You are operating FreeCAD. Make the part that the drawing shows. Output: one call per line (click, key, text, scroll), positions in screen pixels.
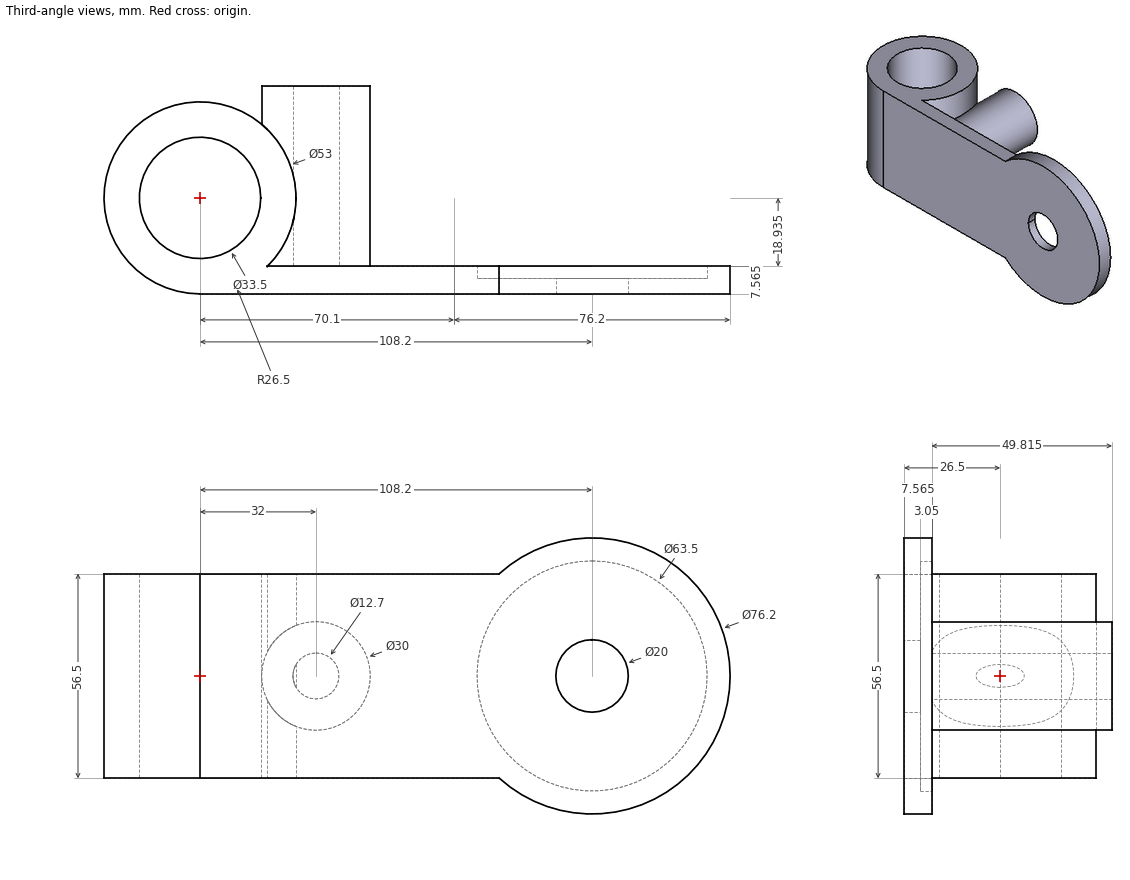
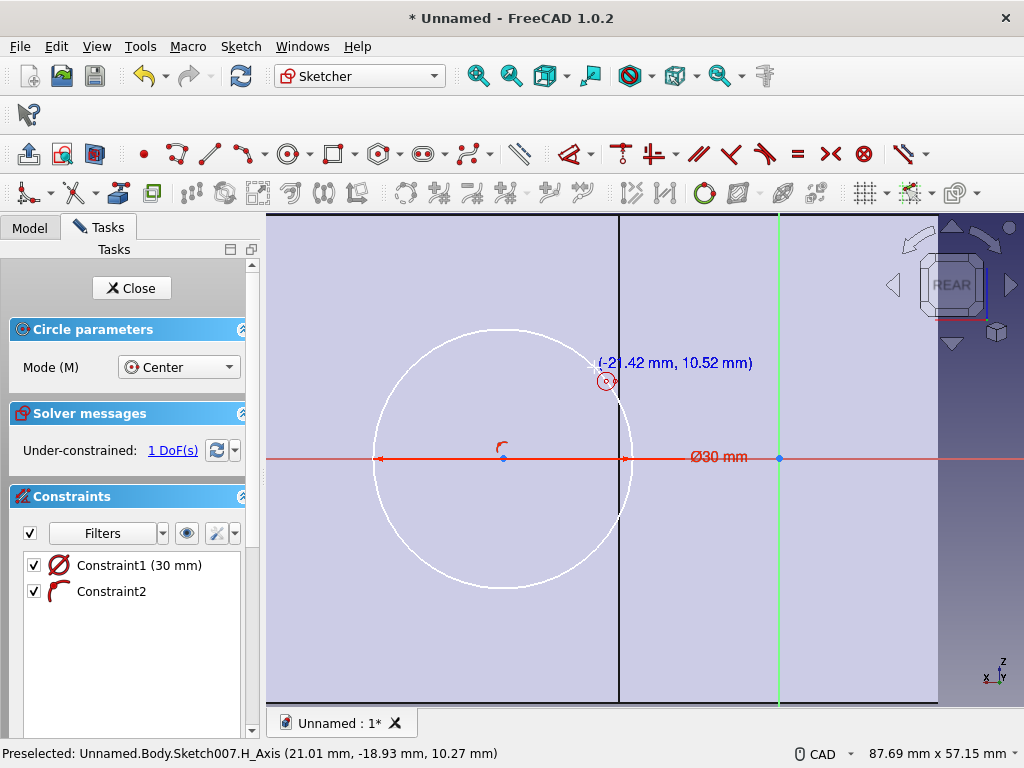
click(503, 459)
move(541, 420)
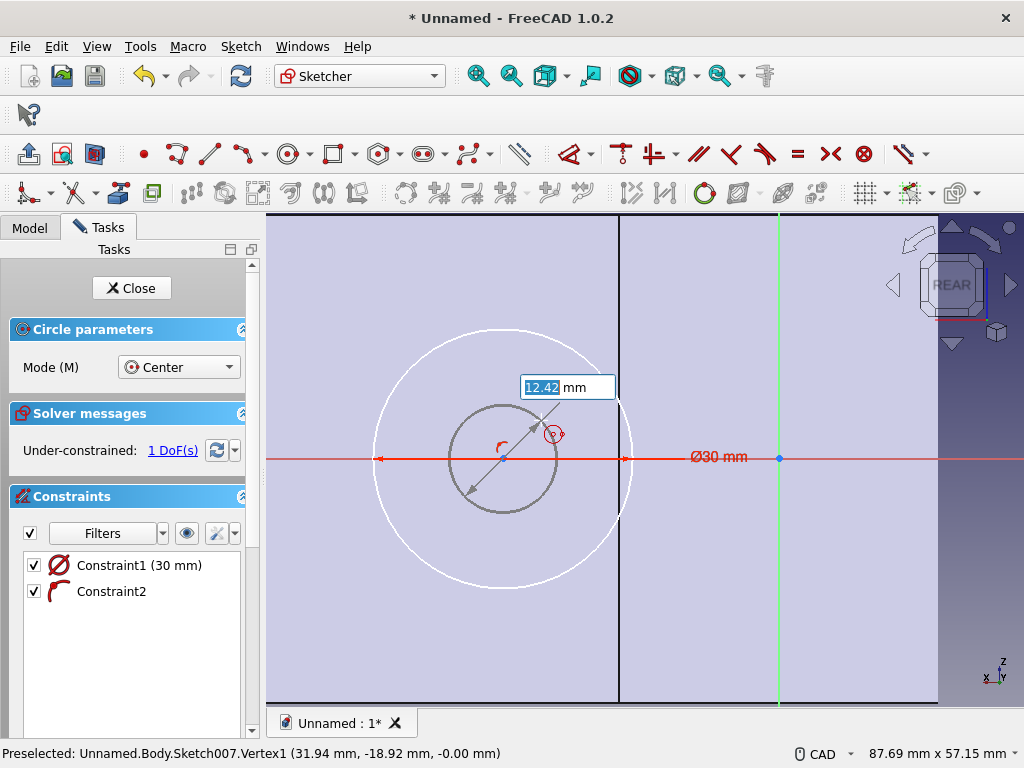
text(12.7)
key(Return)
key(Escape)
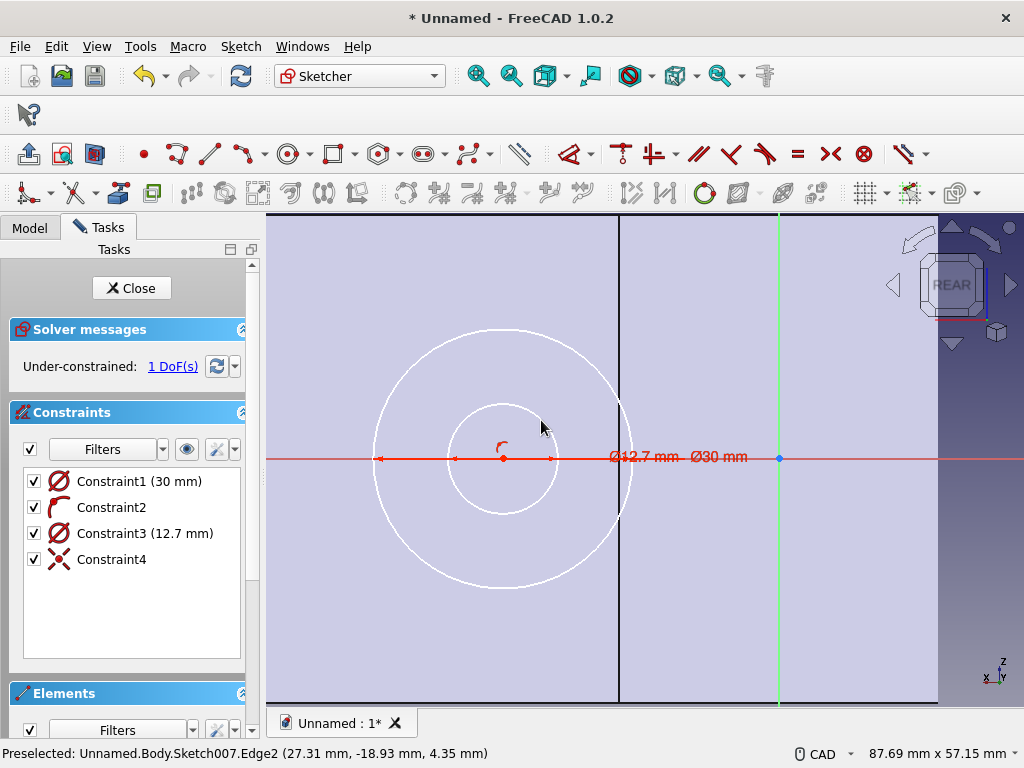
key(d)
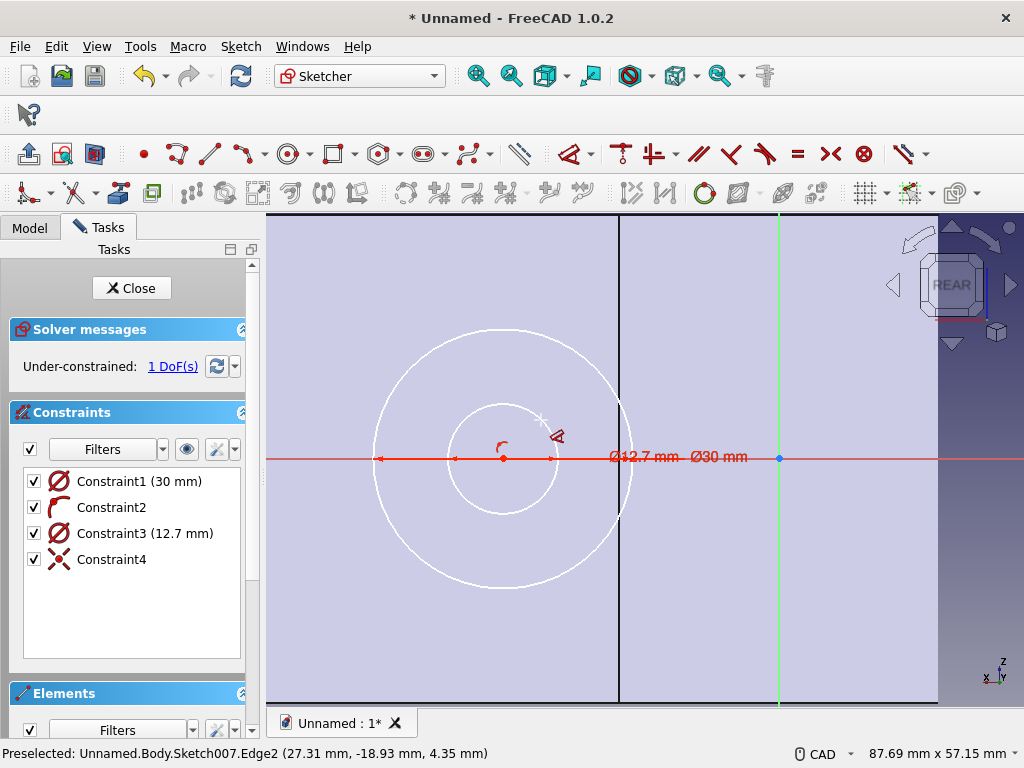
click(503, 459)
click(578, 493)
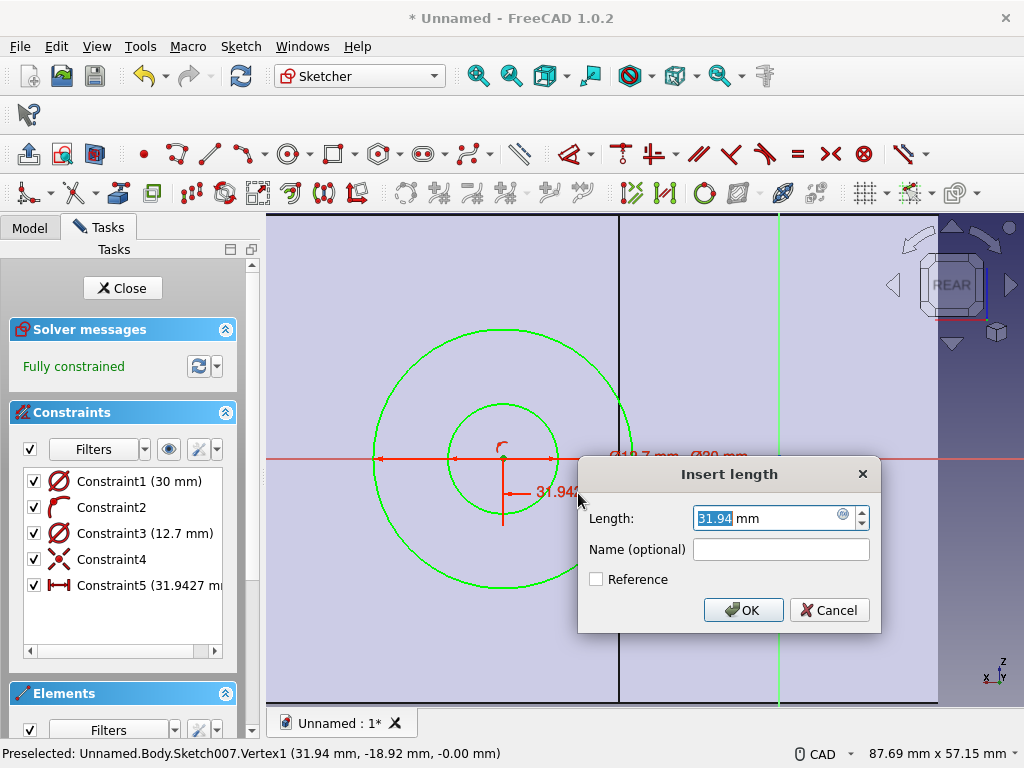
text(32)
key(Return)
key(Escape)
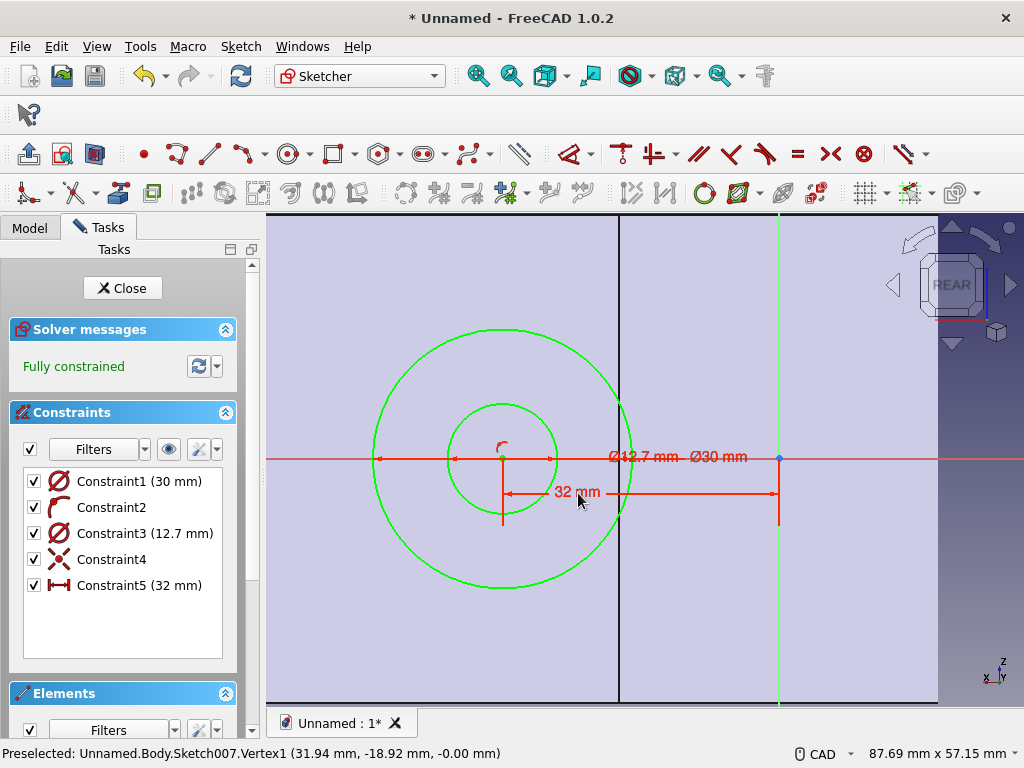
click(123, 288)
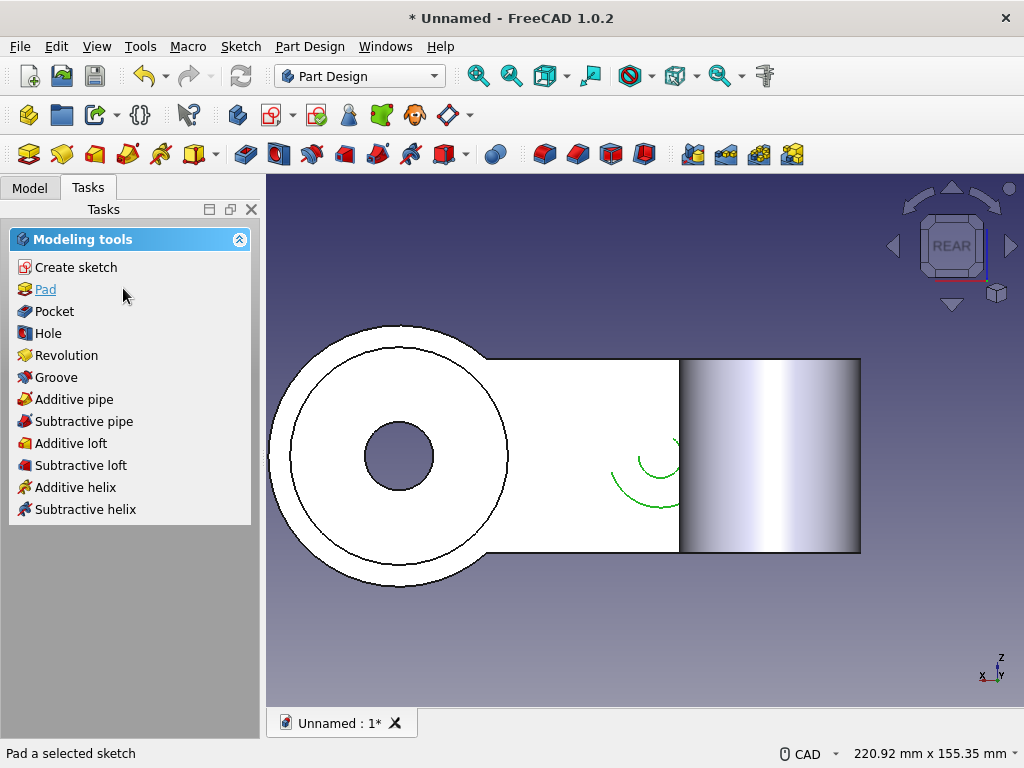
click(29, 154)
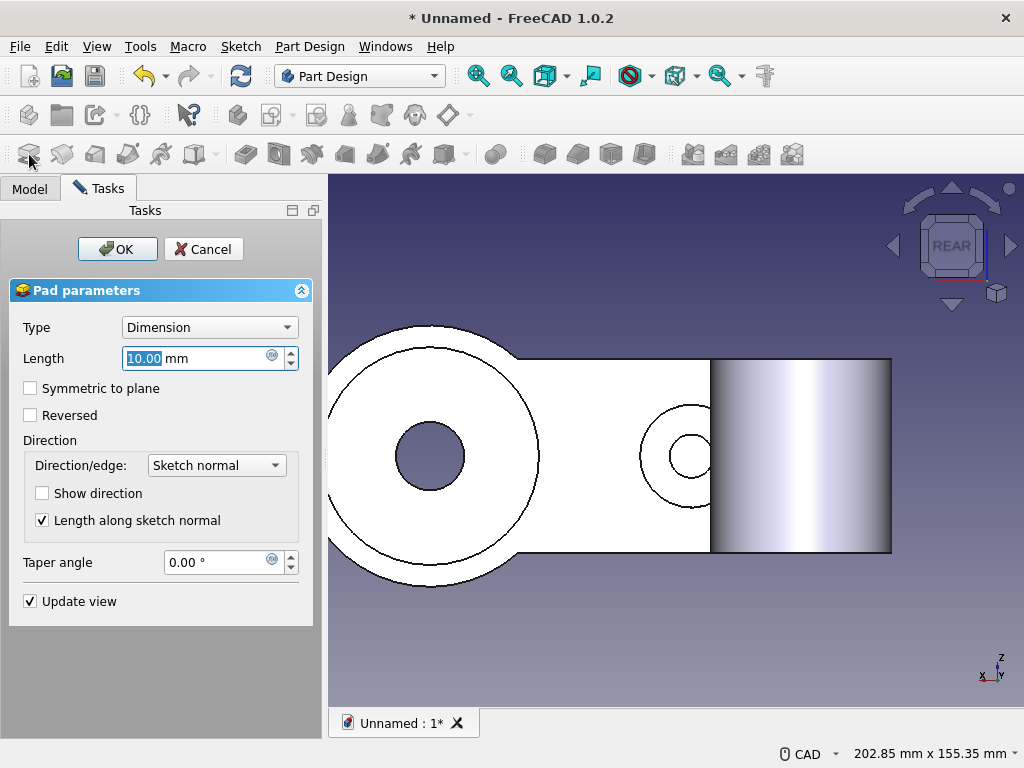
text(49.815)
key(Tab)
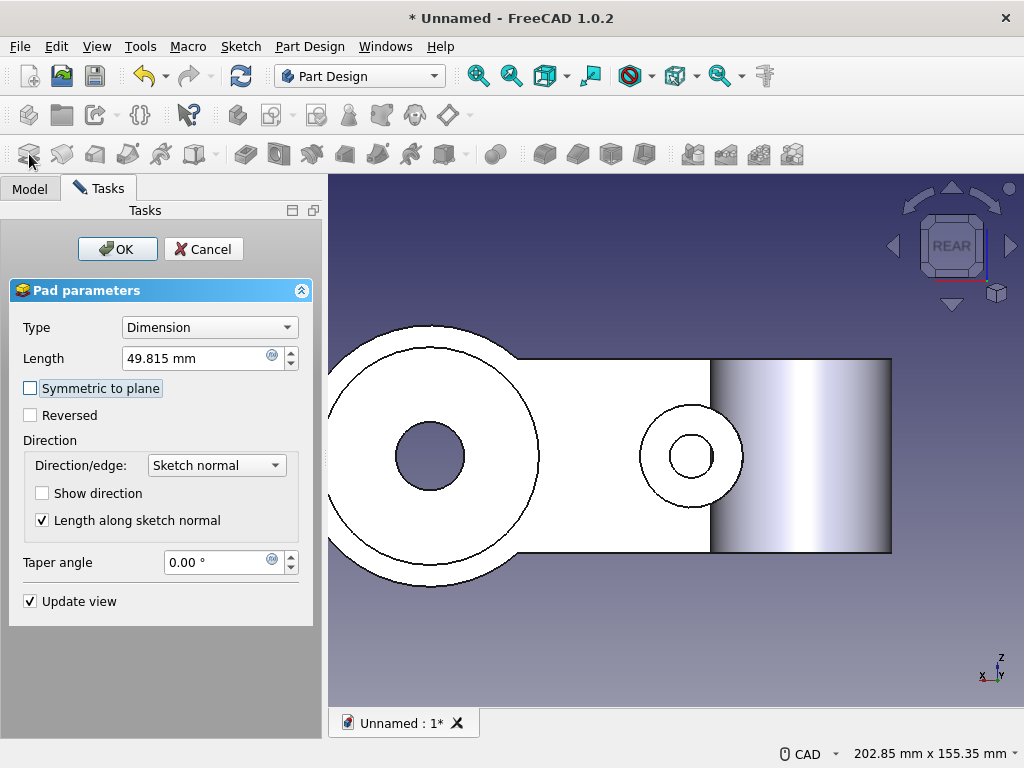
click(118, 249)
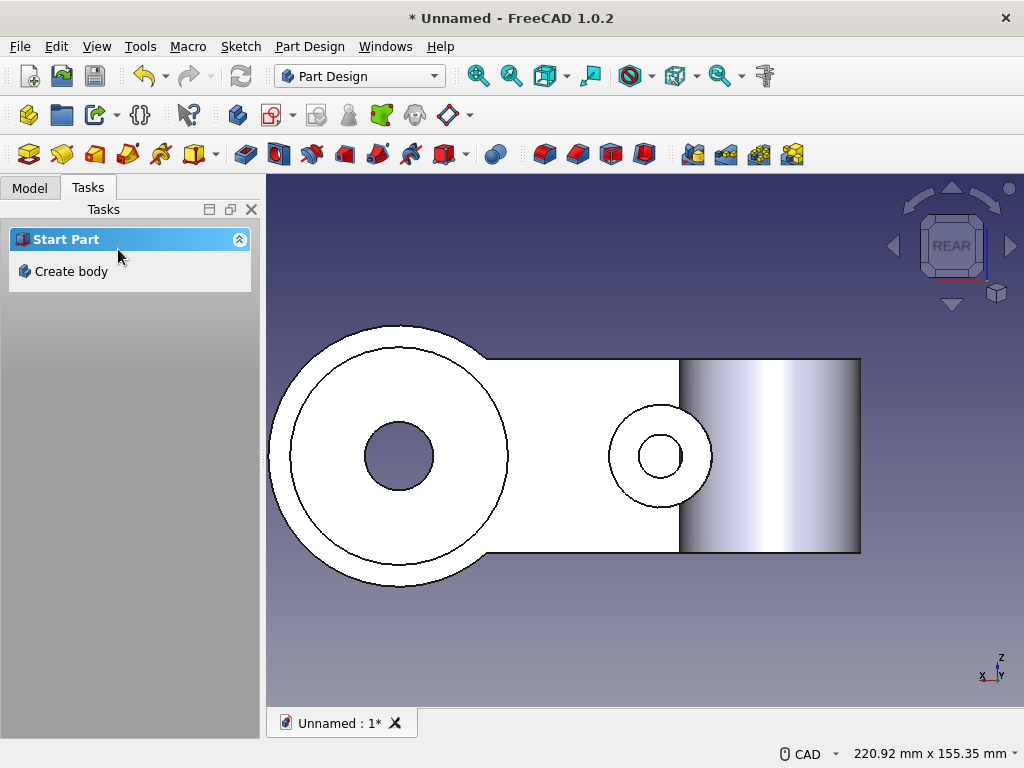
key(0)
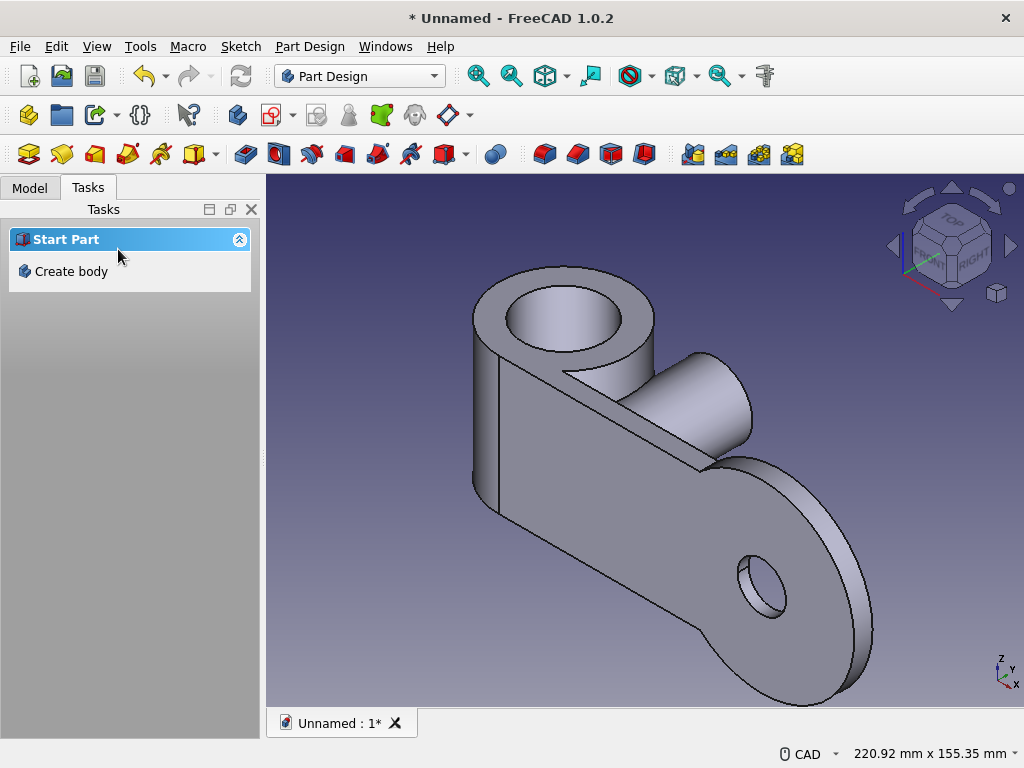
click(479, 76)